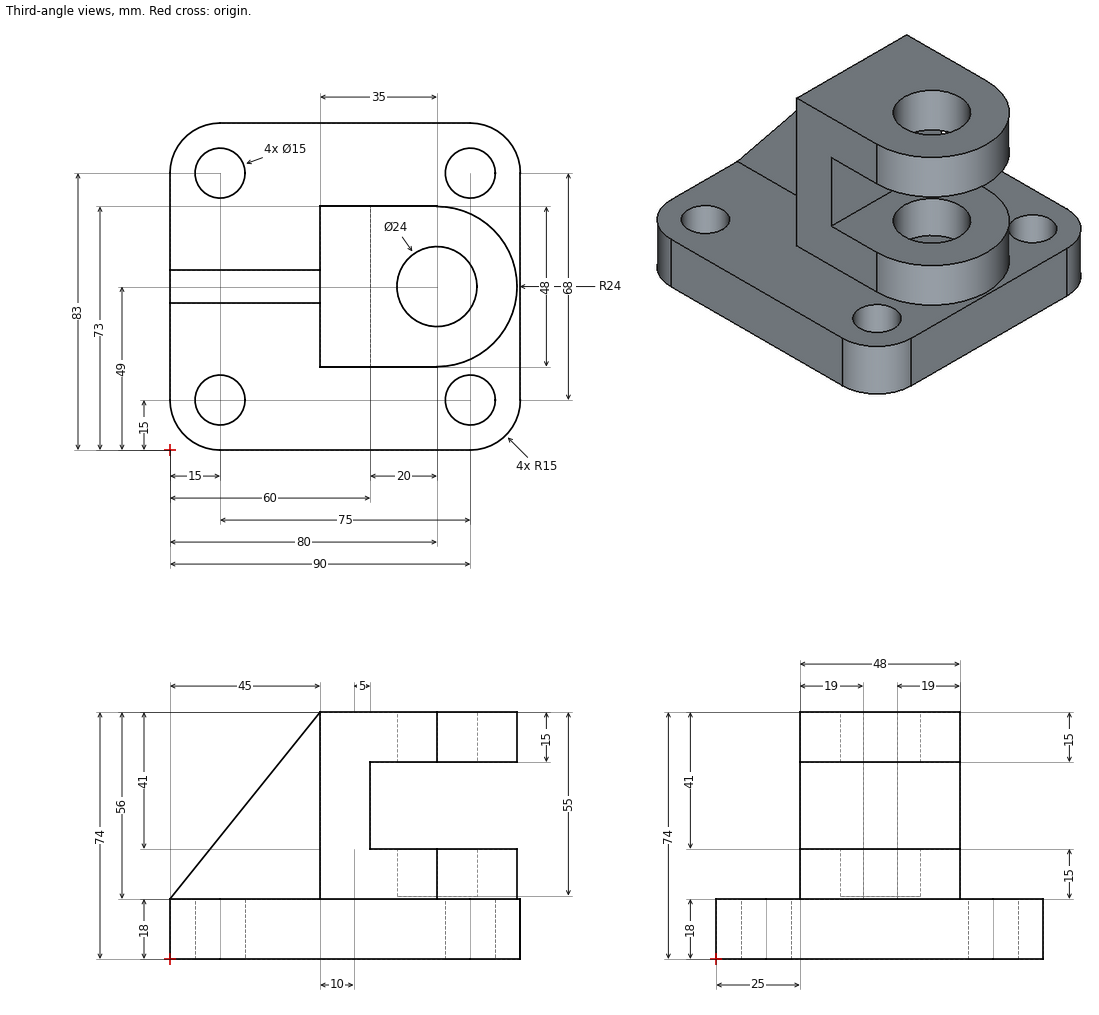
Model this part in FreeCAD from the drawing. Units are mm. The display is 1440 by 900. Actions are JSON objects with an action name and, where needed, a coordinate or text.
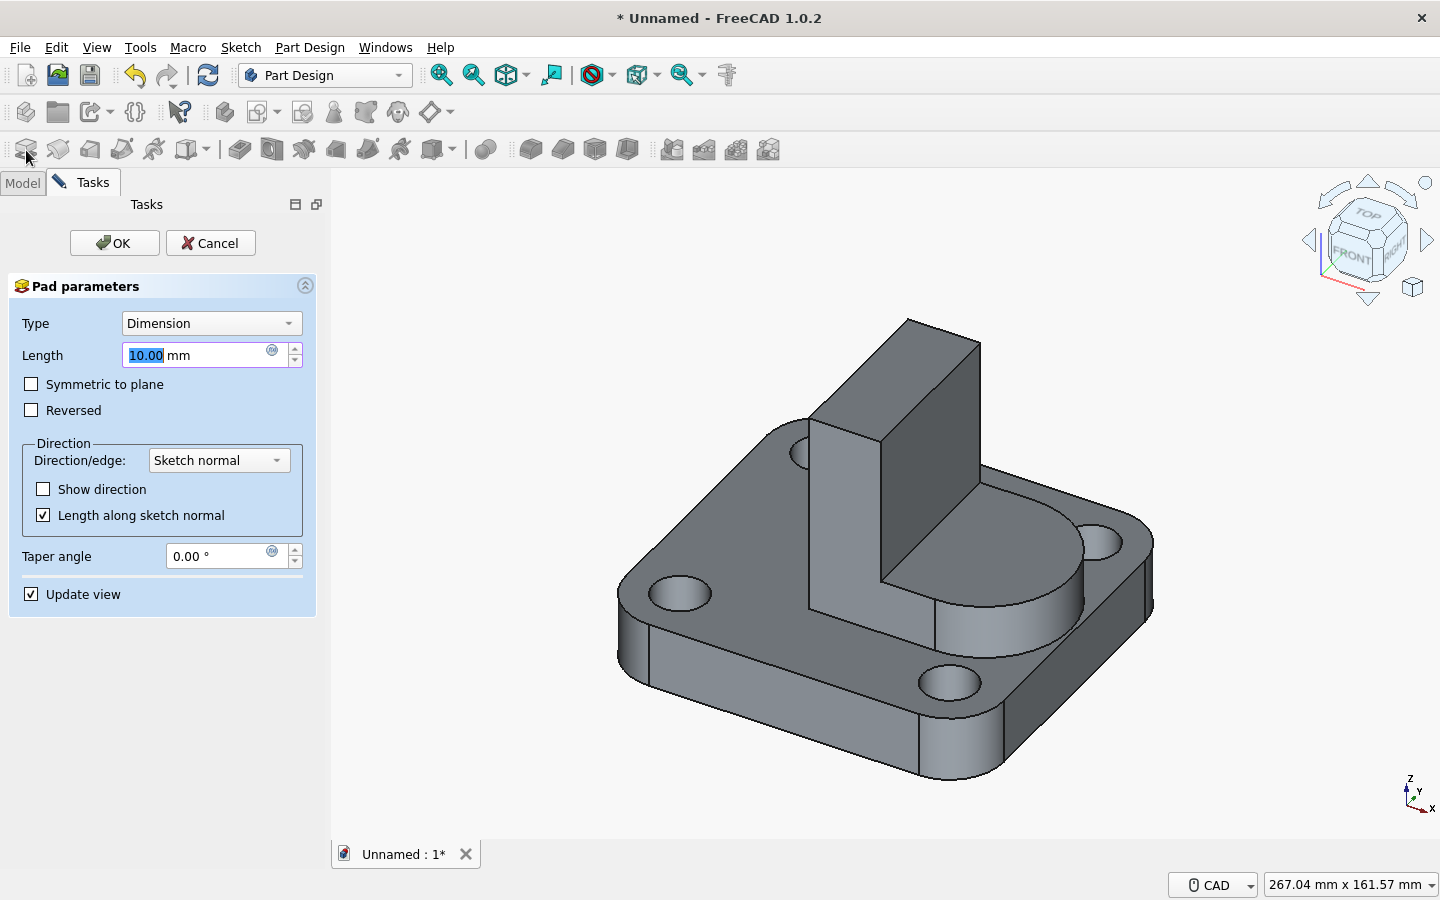
{"action": "type", "text": "5"}
{"action": "key", "text": "Tab"}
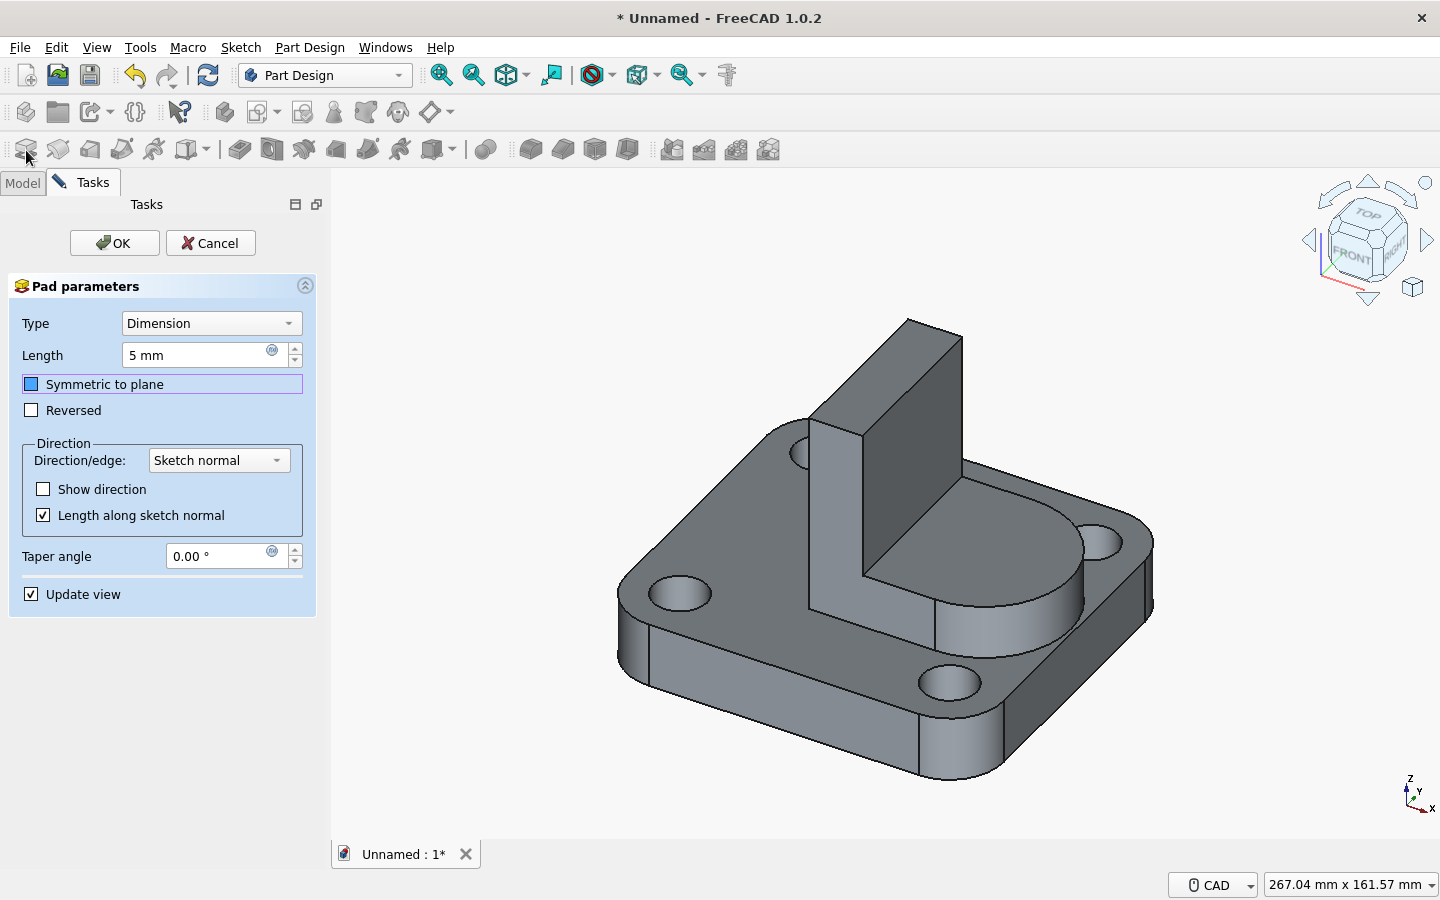
{"action": "left_click", "coordinate": [115, 243]}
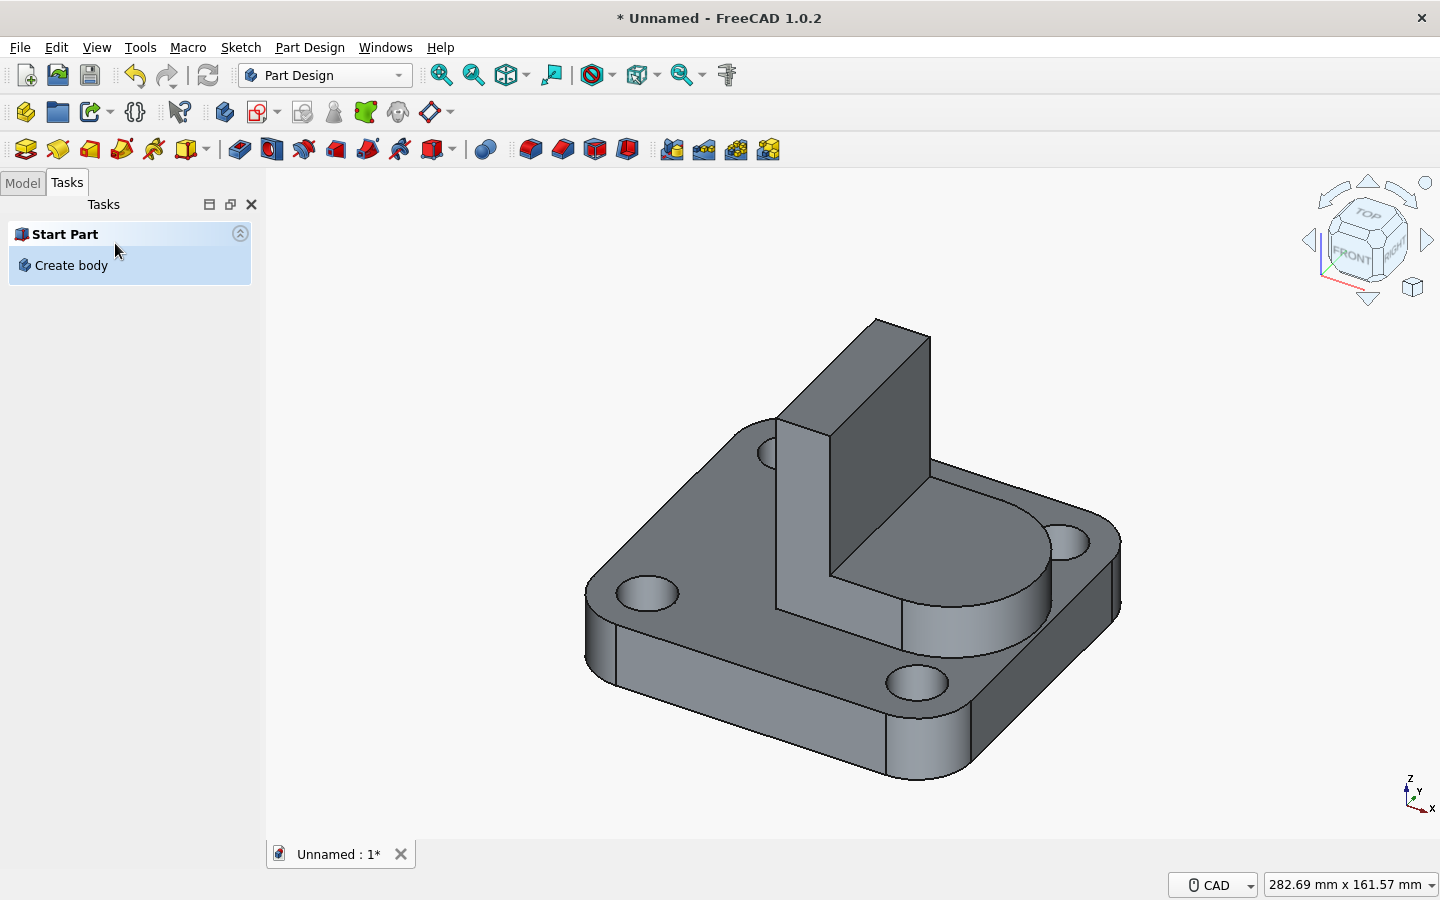
{"action": "left_click", "coordinate": [881, 348]}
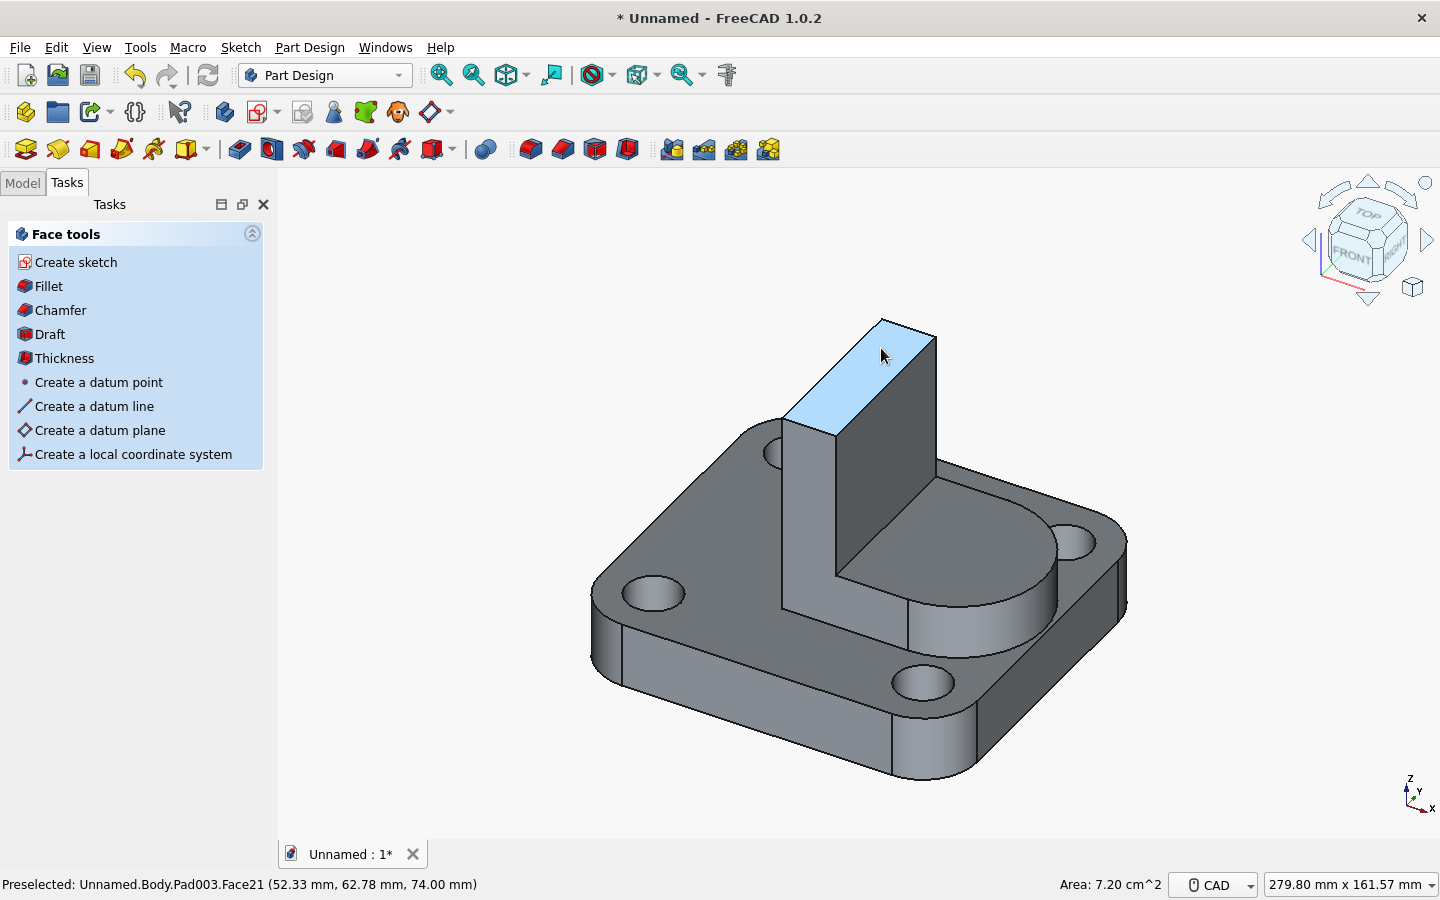
{"action": "left_click", "coordinate": [258, 112]}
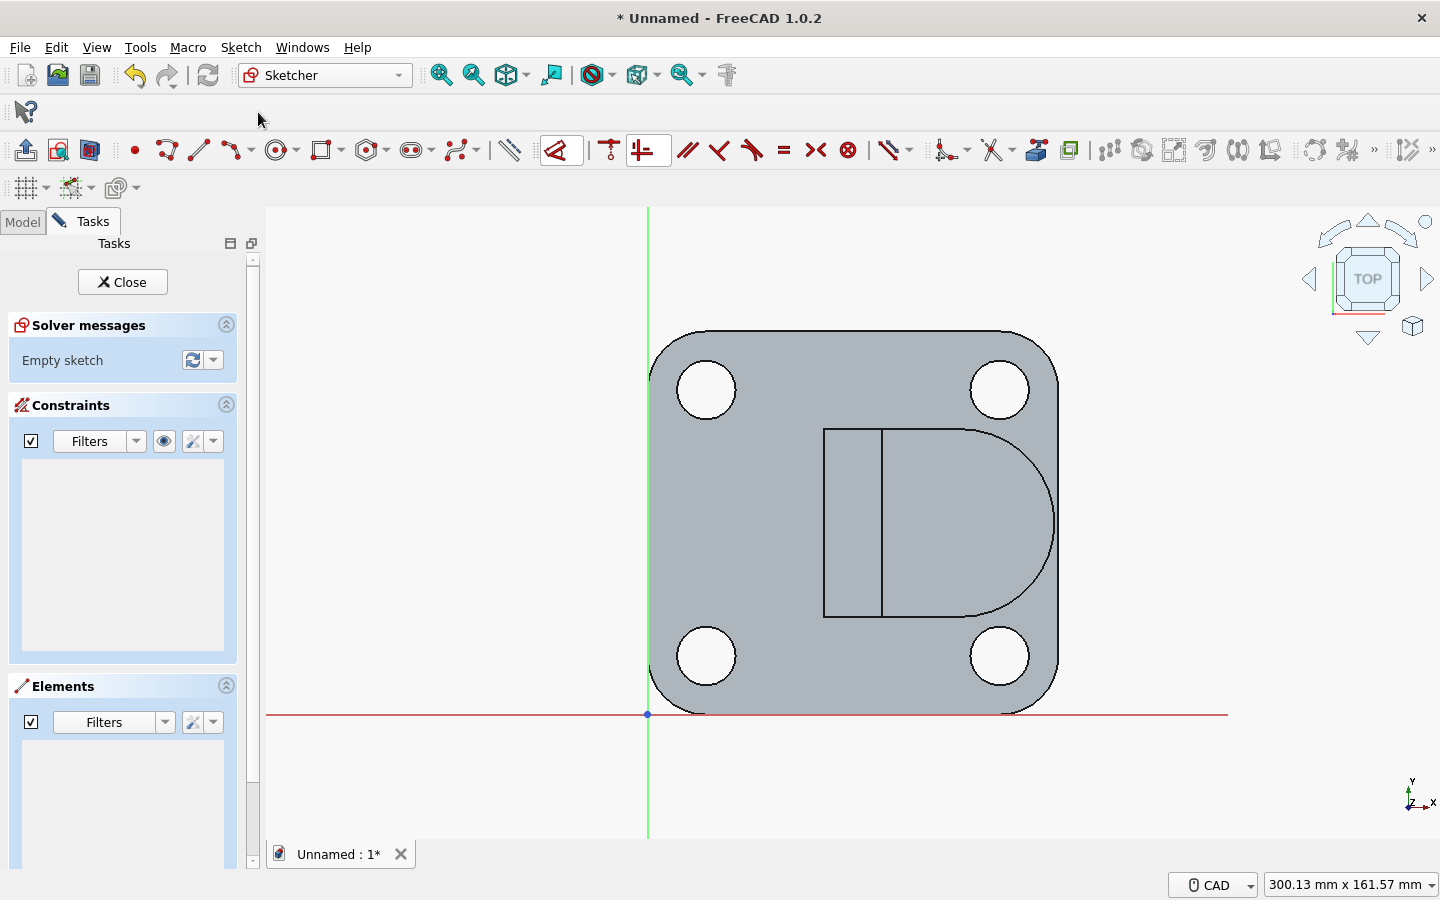
{"action": "scroll", "coordinate": [844, 671], "scroll_direction": "up", "scroll_amount": 2}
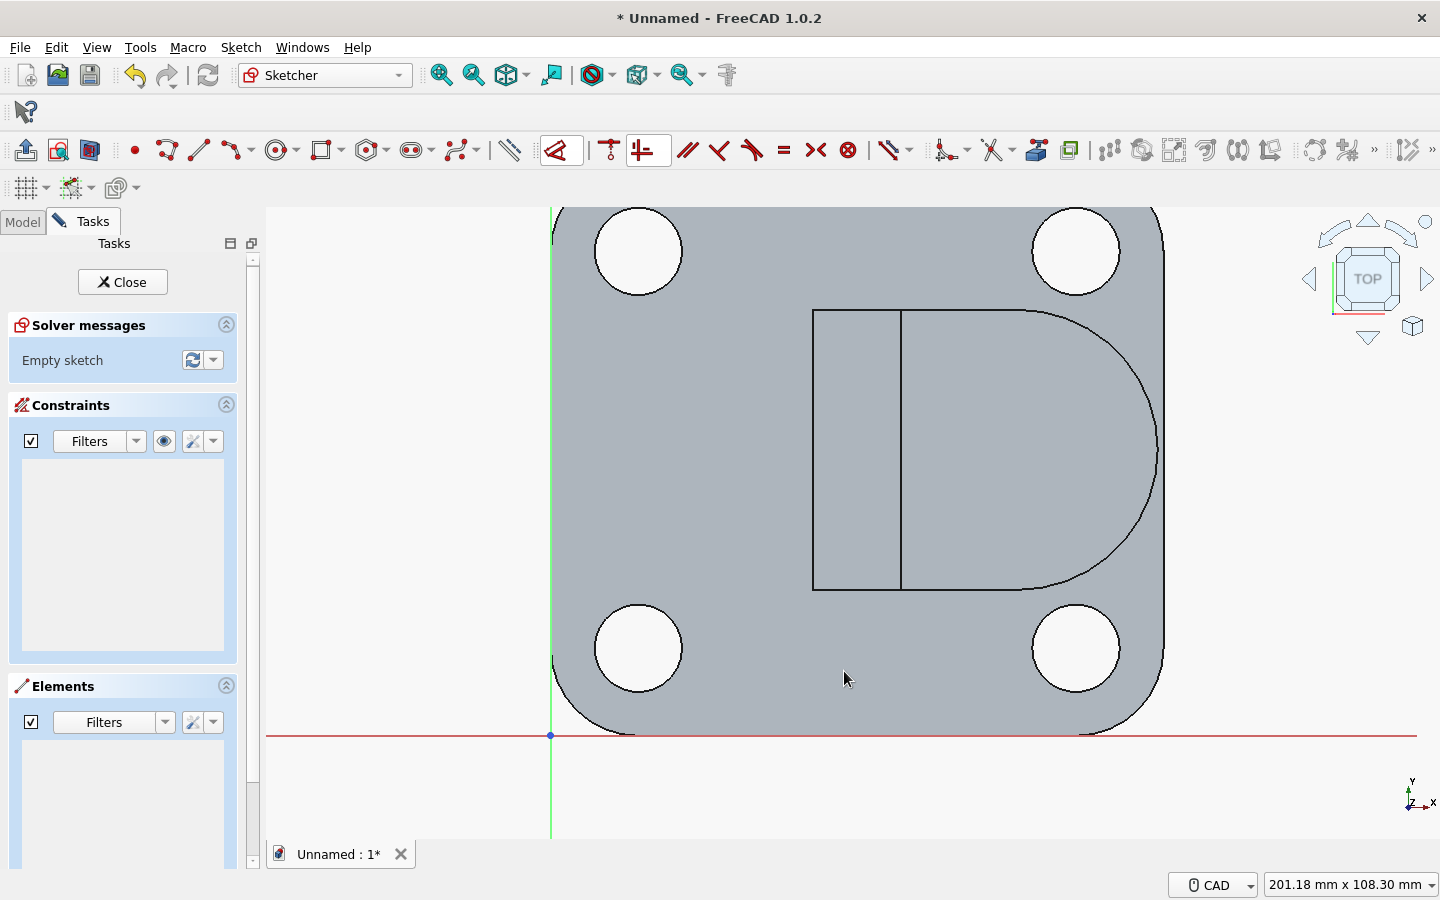
{"action": "left_click", "coordinate": [322, 150]}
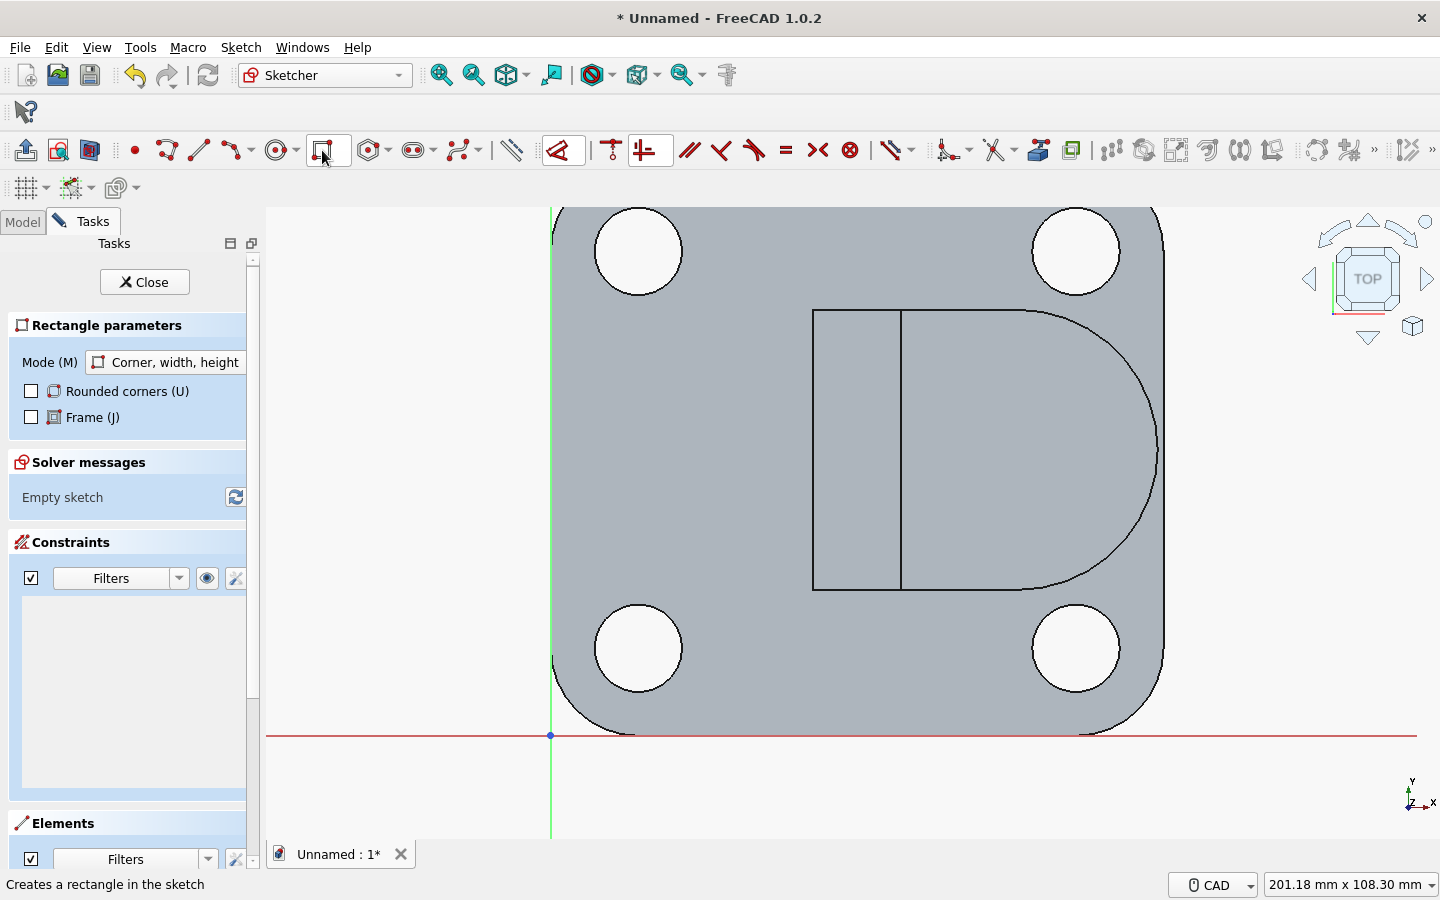
{"action": "left_click", "coordinate": [901, 310]}
{"action": "left_click", "coordinate": [1018, 590]}
{"action": "key", "text": "Escape"}